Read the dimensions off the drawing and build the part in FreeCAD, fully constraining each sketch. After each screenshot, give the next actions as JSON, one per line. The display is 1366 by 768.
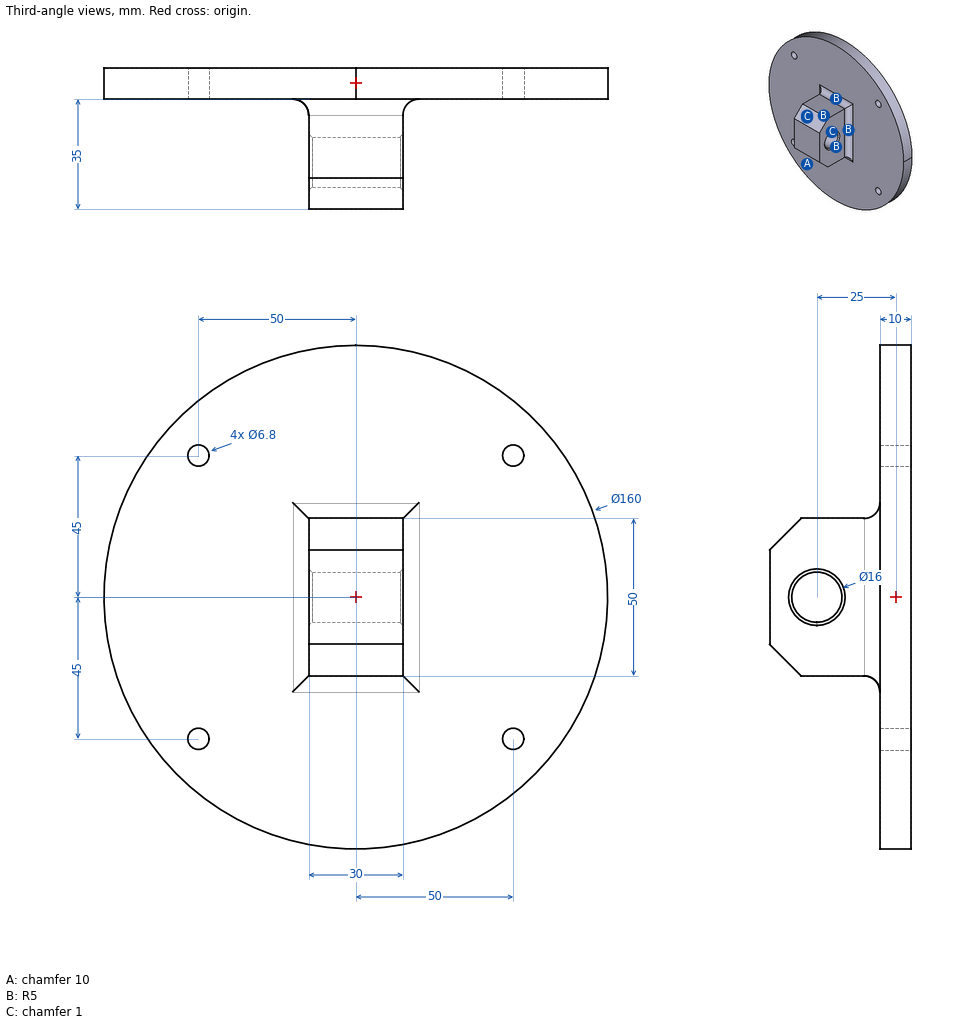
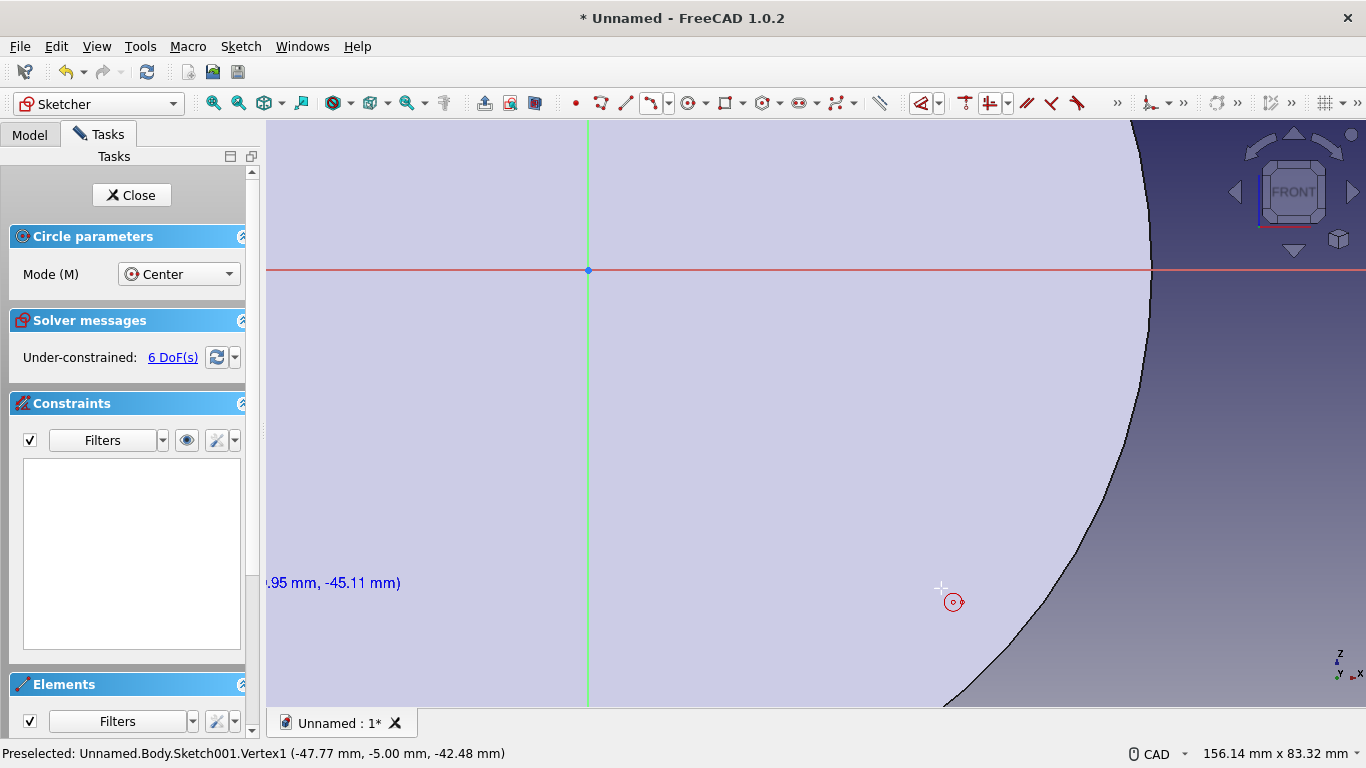
{"action": "left_click", "coordinate": [941, 587]}
{"action": "left_click", "coordinate": [958, 570]}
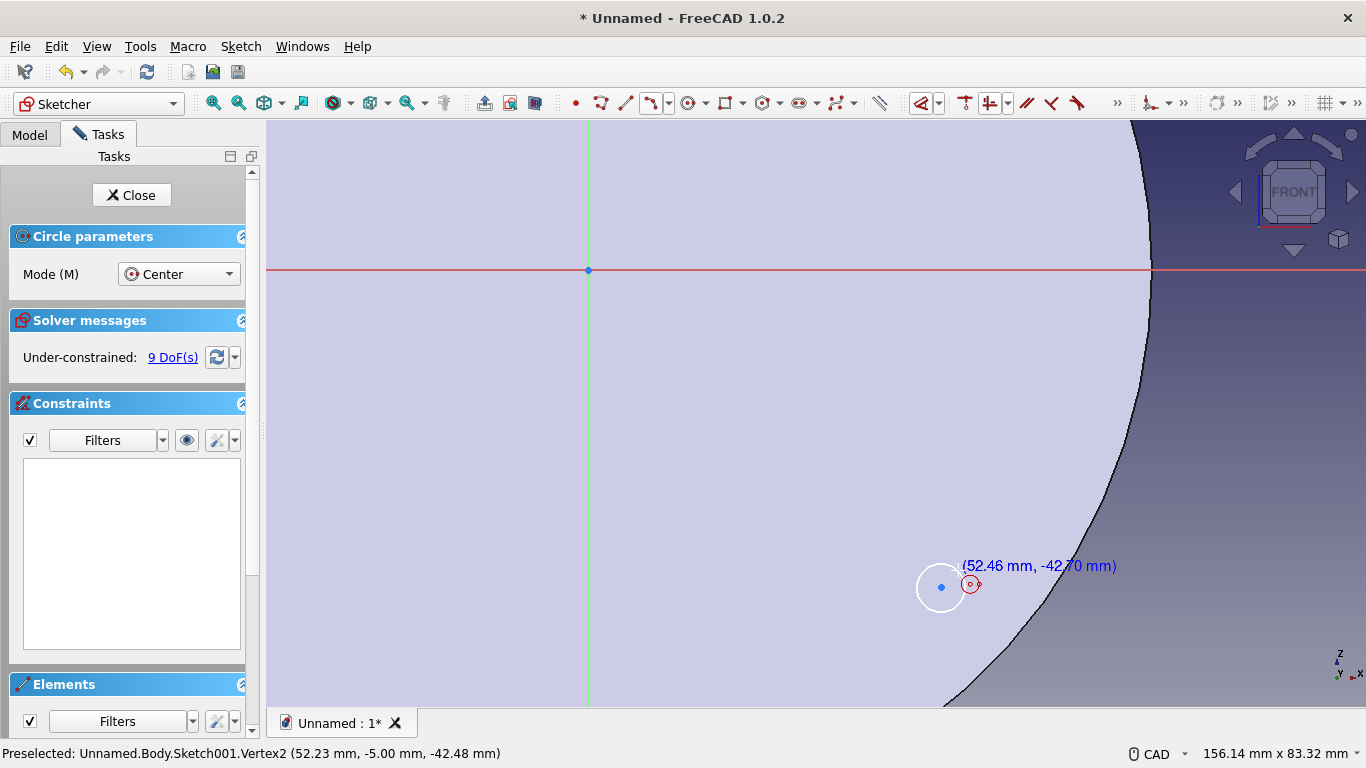
{"action": "scroll", "coordinate": [941, 588], "scroll_direction": "down", "scroll_amount": 3}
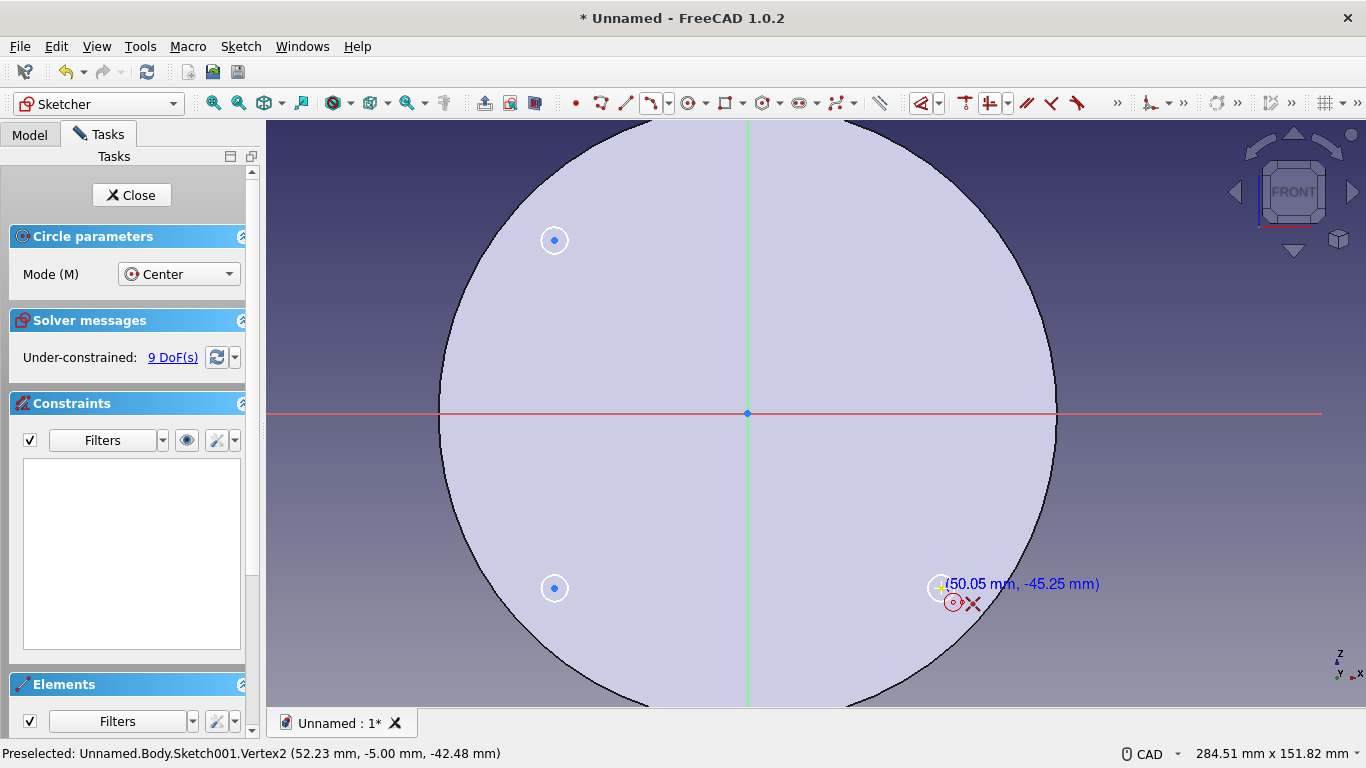
{"action": "scroll", "coordinate": [941, 240], "scroll_direction": "up", "scroll_amount": 3}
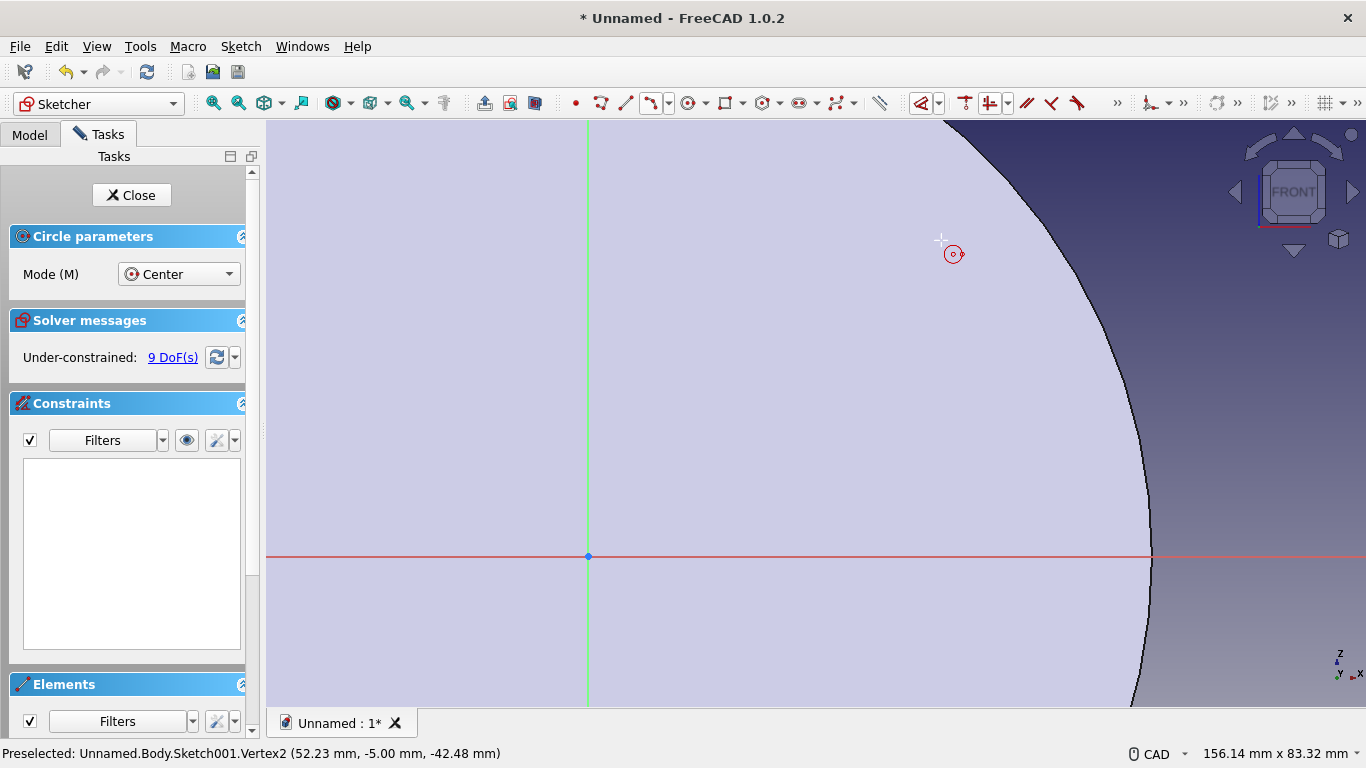
{"action": "left_click", "coordinate": [941, 240]}
{"action": "left_click", "coordinate": [958, 223]}
{"action": "key", "text": "Escape"}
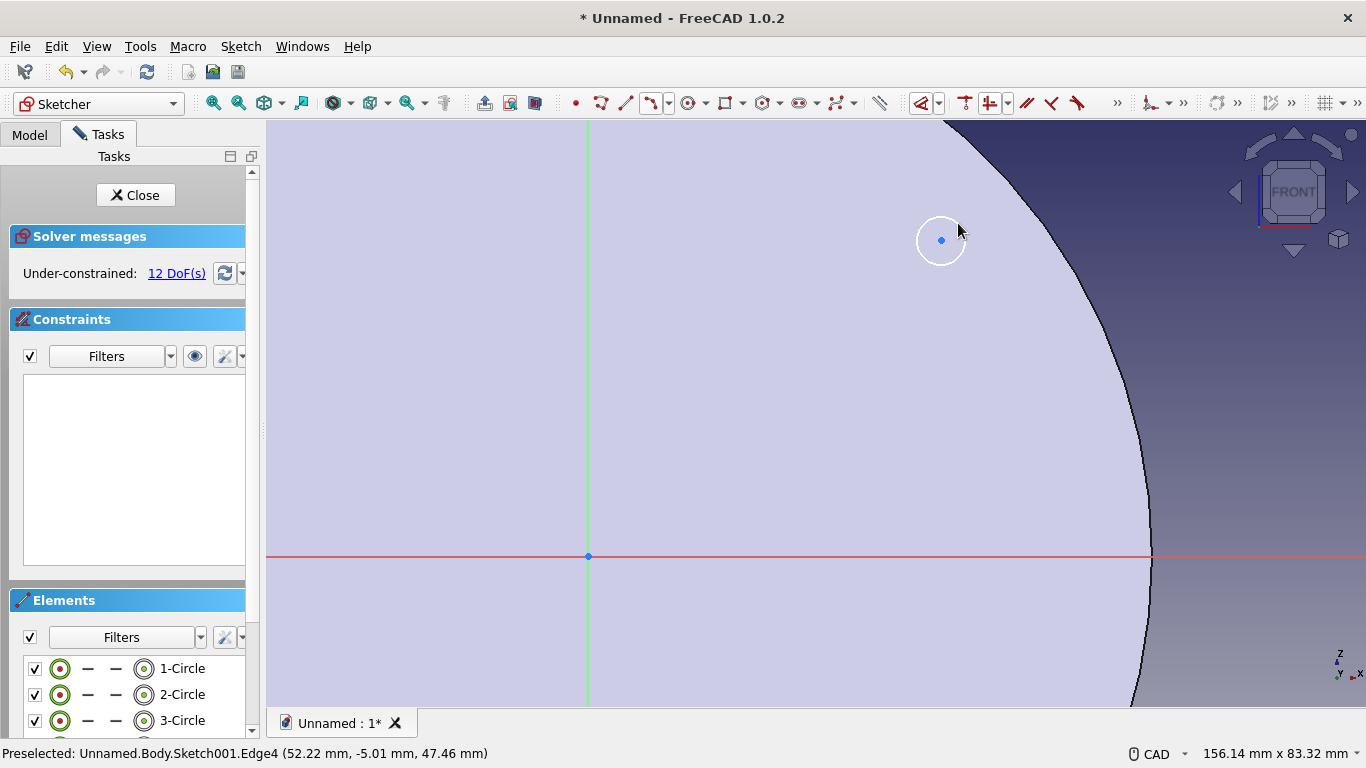
{"action": "scroll", "coordinate": [941, 239], "scroll_direction": "down", "scroll_amount": 3}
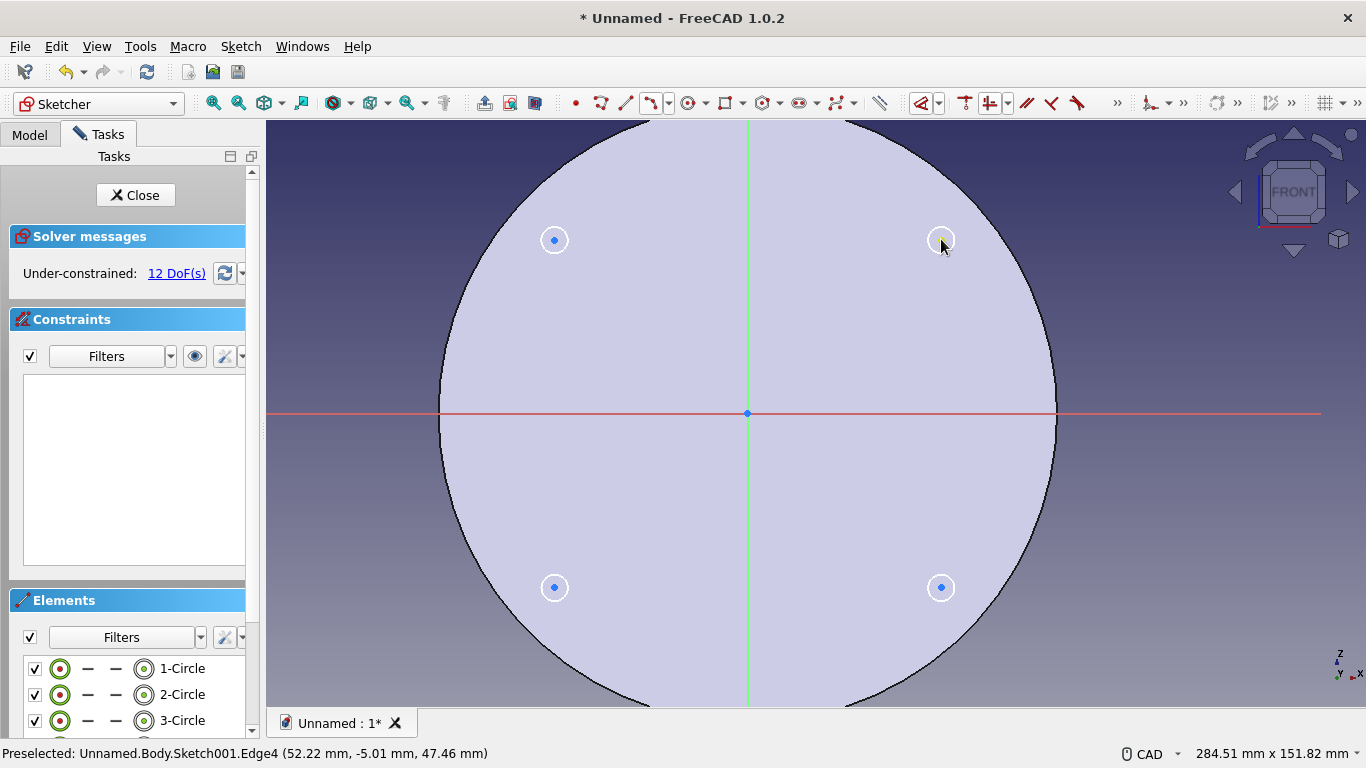
{"action": "left_click", "coordinate": [564, 231]}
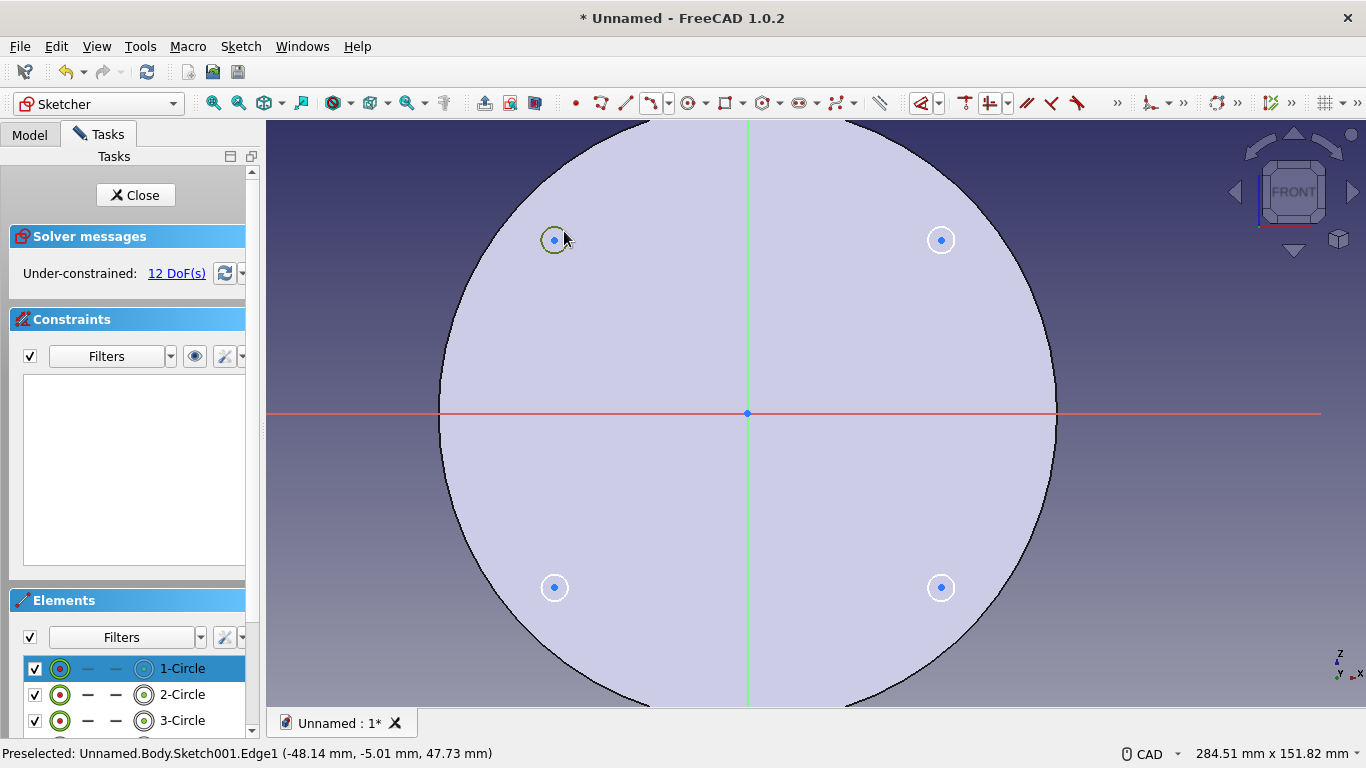
{"action": "left_click", "coordinate": [564, 579]}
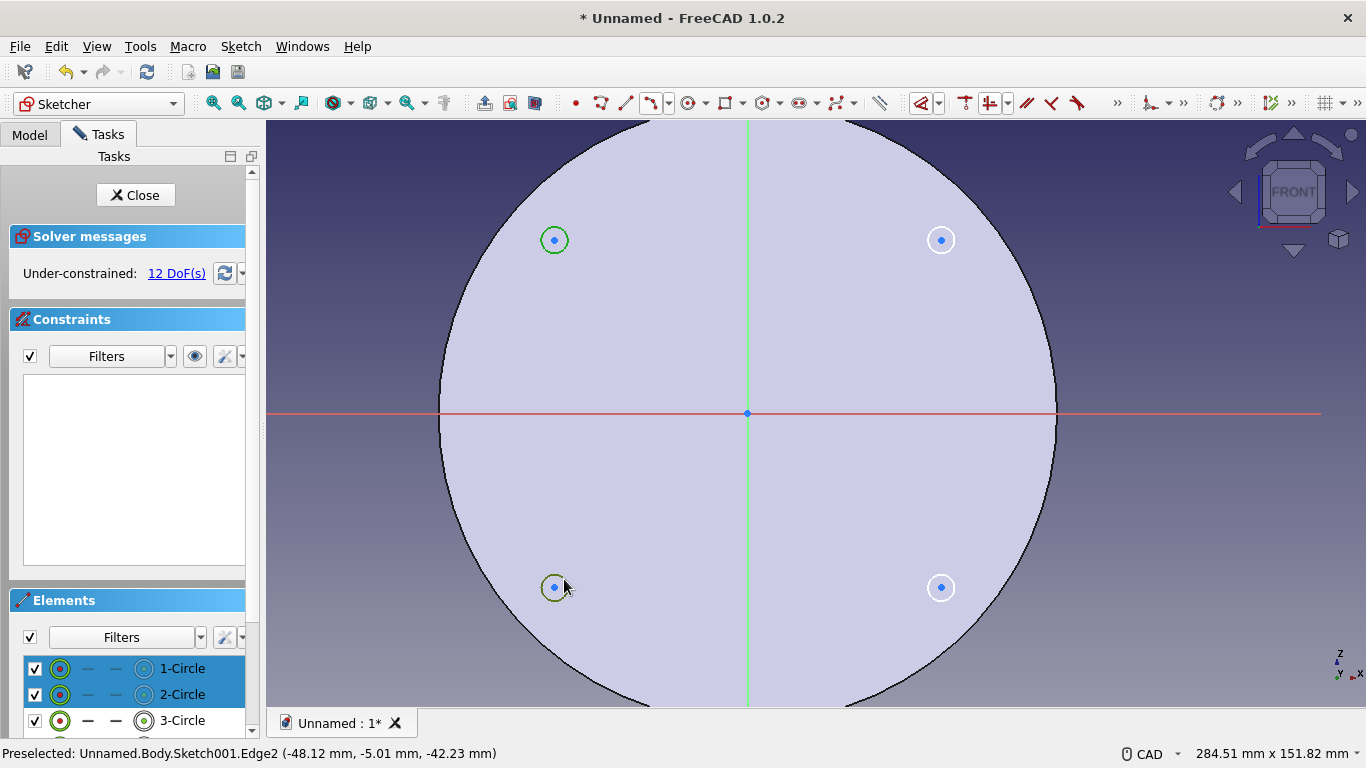
{"action": "left_click", "coordinate": [951, 579]}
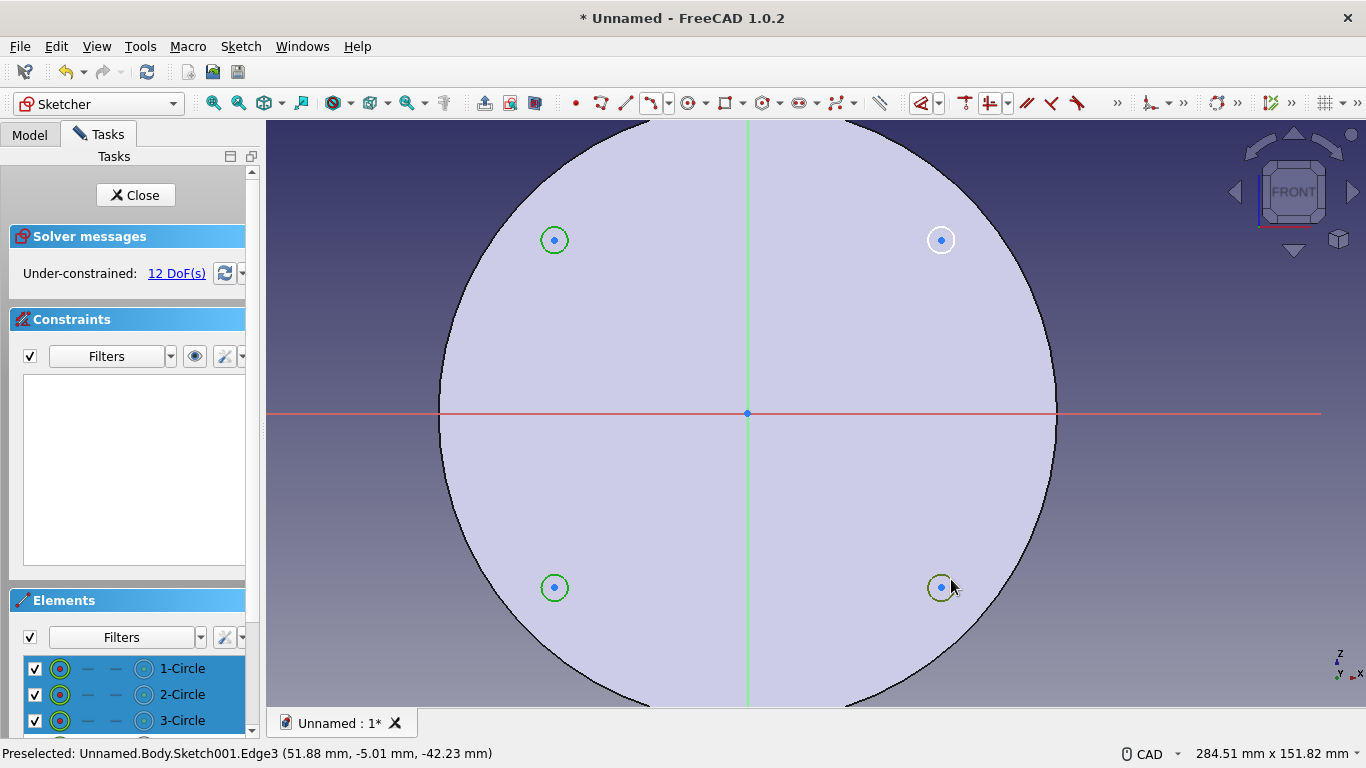
{"action": "left_click", "coordinate": [951, 231]}